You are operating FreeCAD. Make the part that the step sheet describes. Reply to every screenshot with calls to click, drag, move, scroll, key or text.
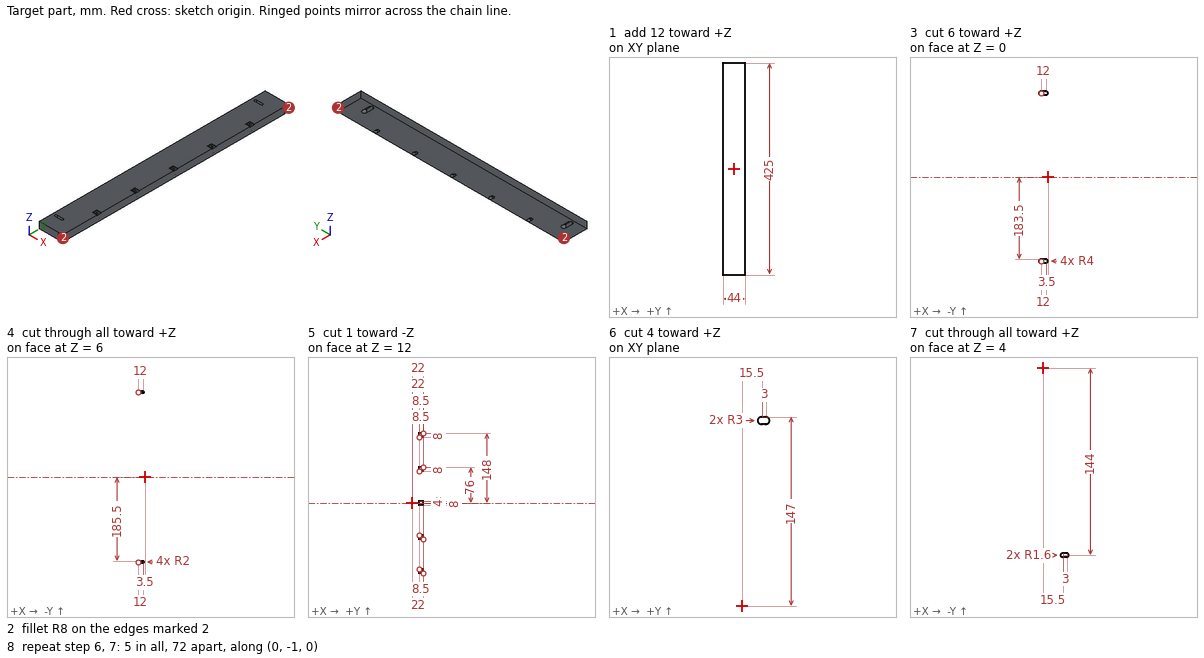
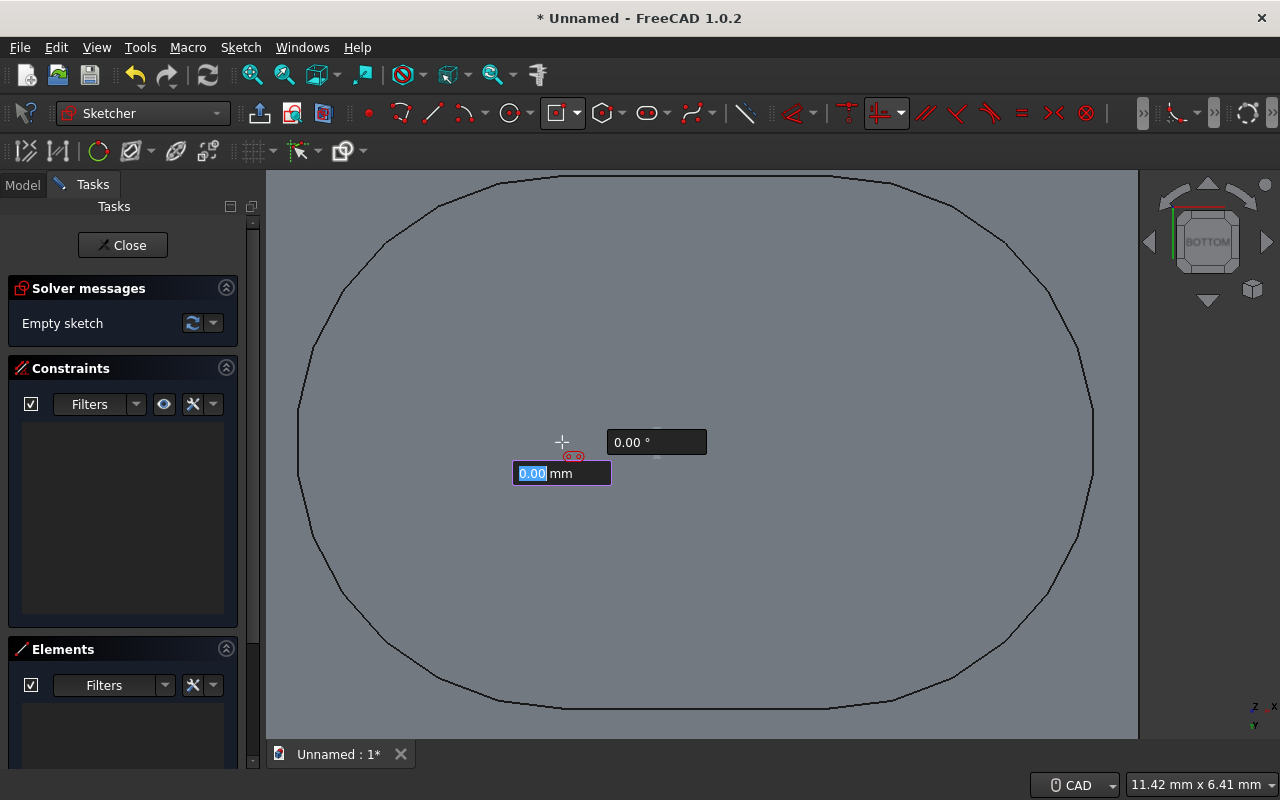
click(829, 442)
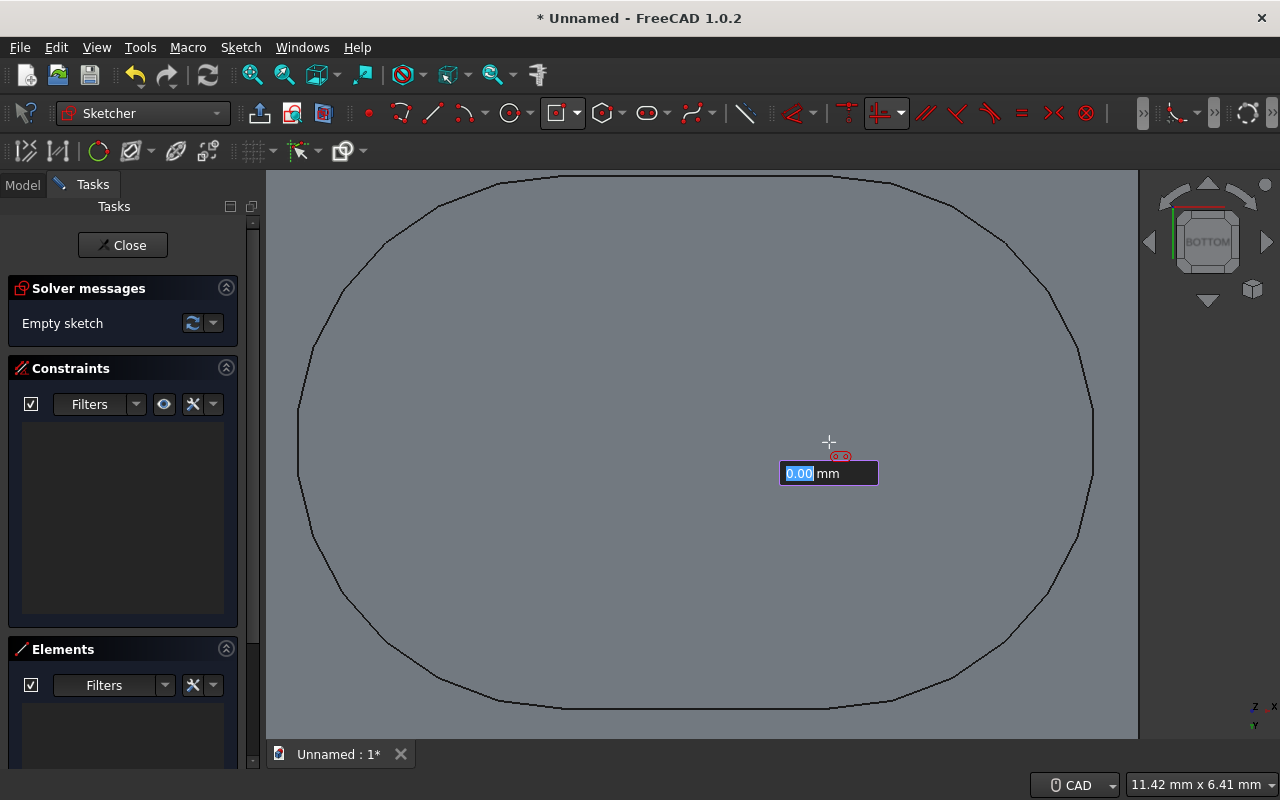
click(695, 584)
key(Escape)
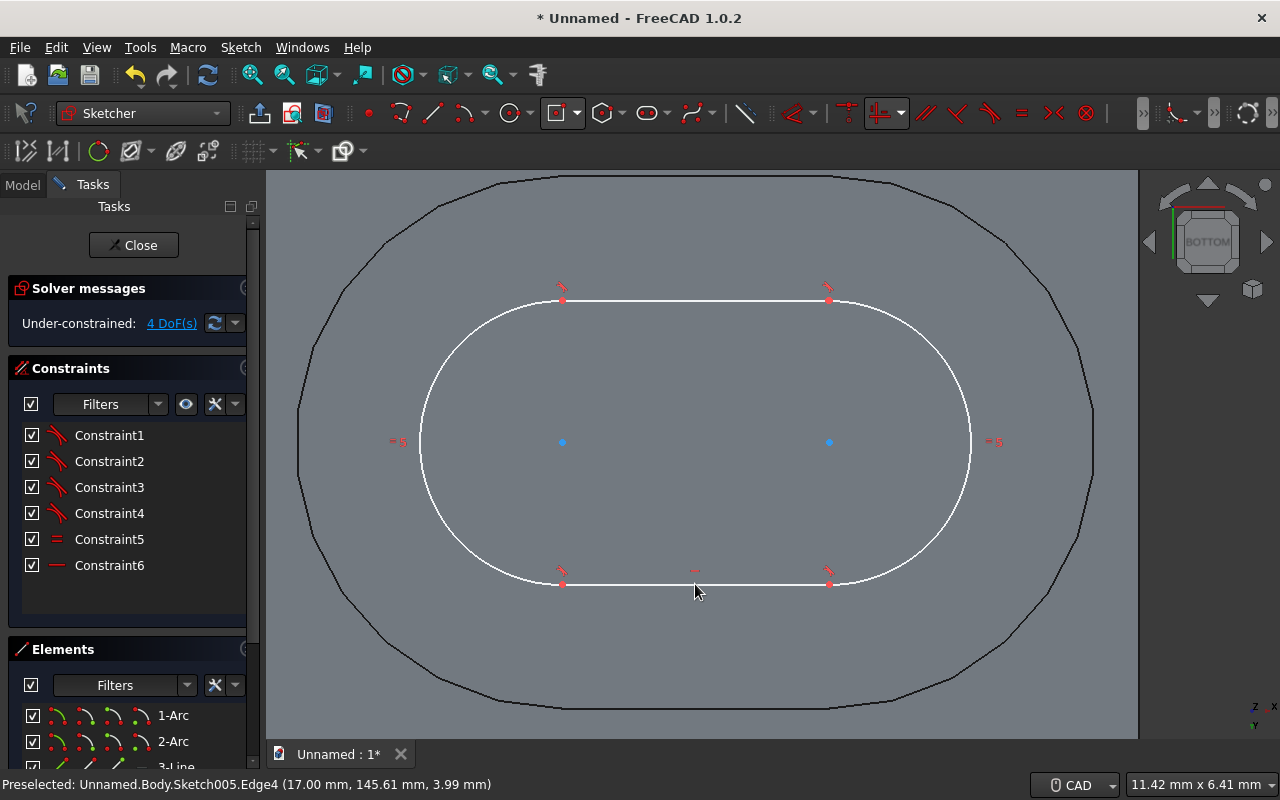
click(792, 114)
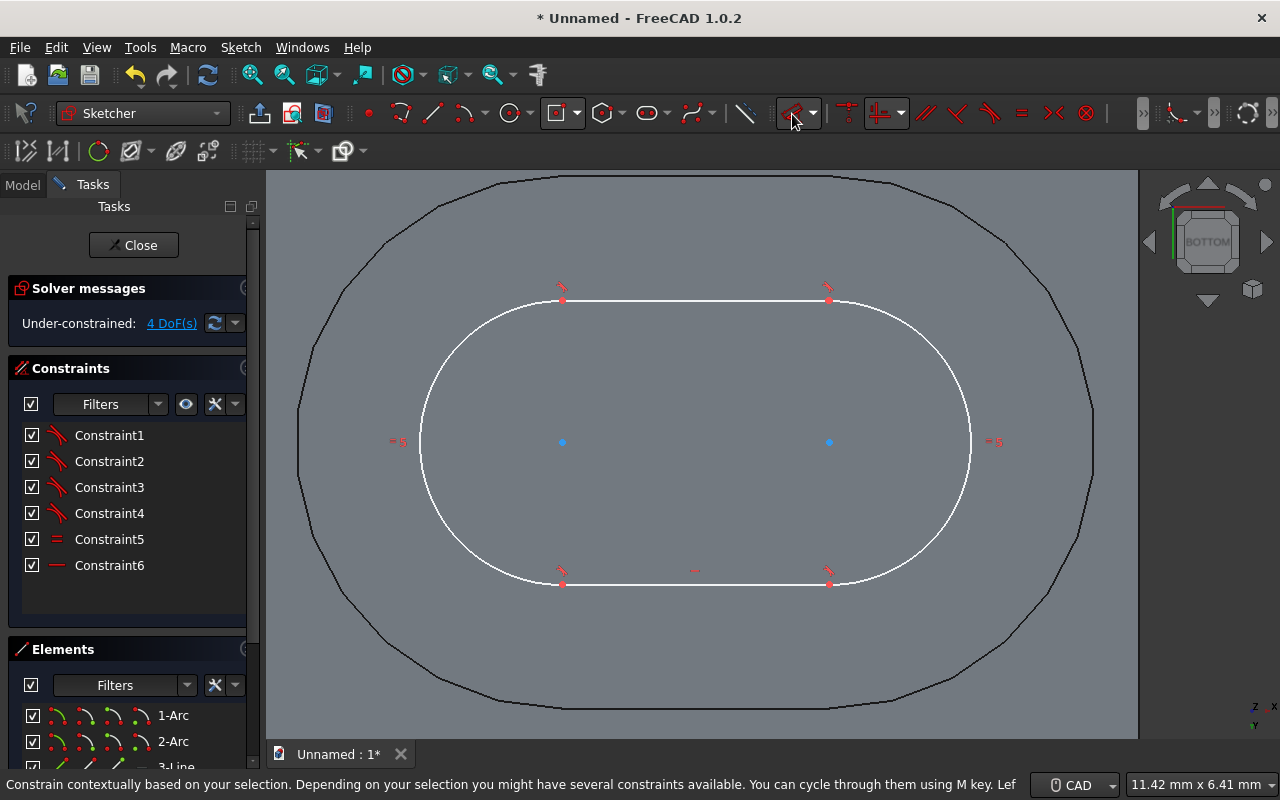
click(447, 360)
click(421, 341)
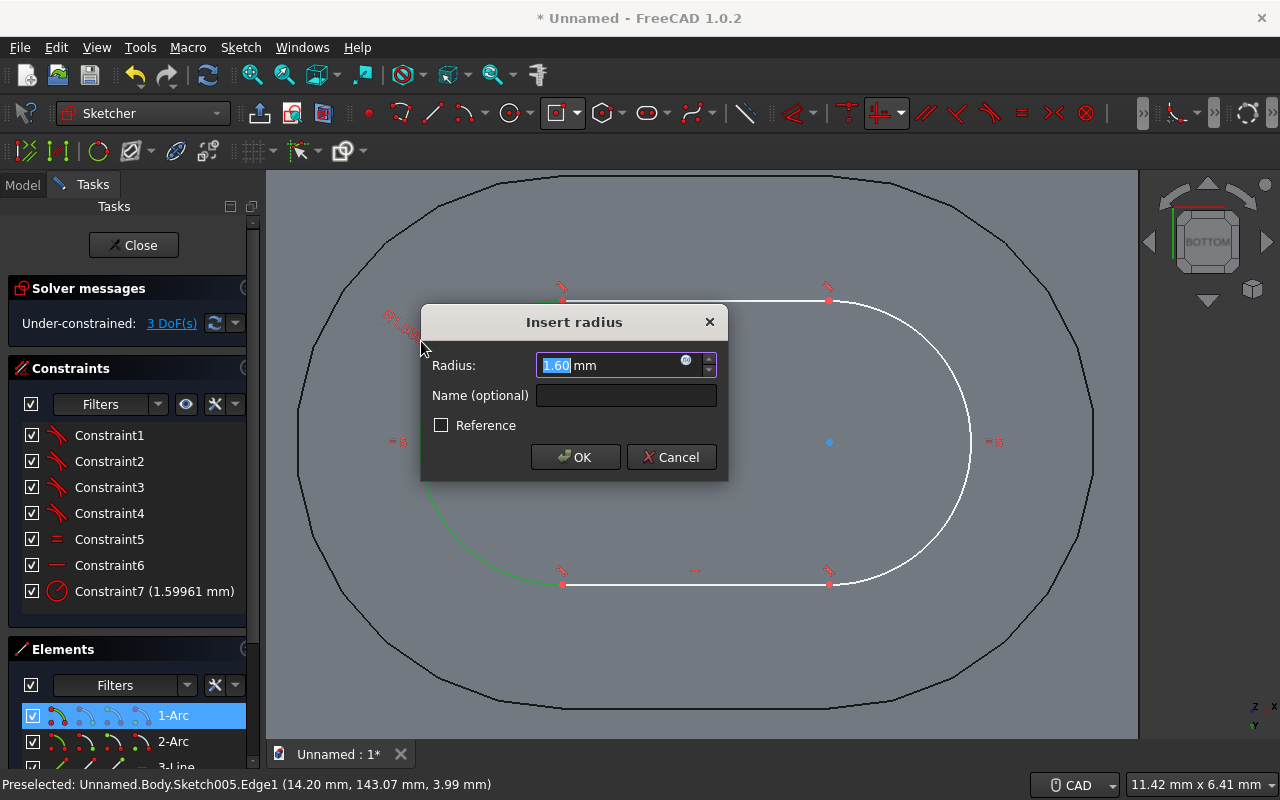
text(1.6)
key(Return)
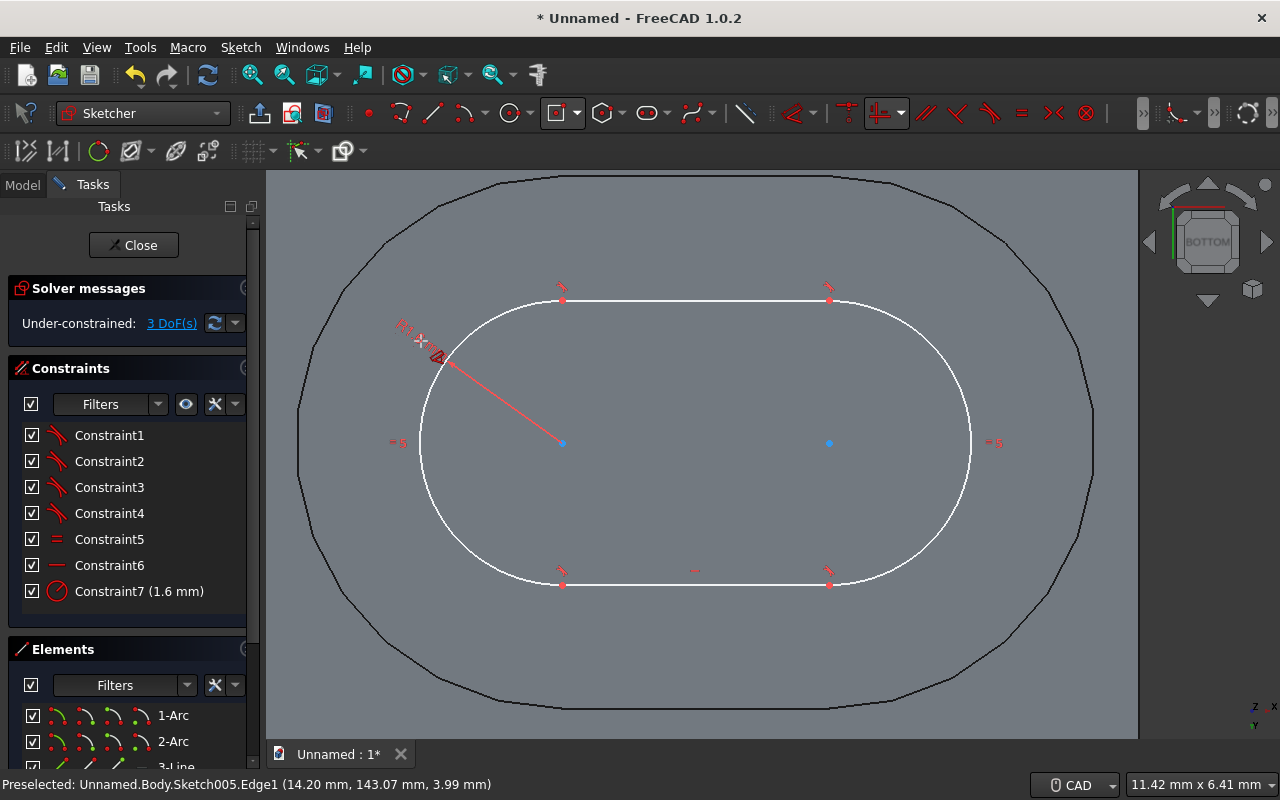
click(642, 301)
click(695, 267)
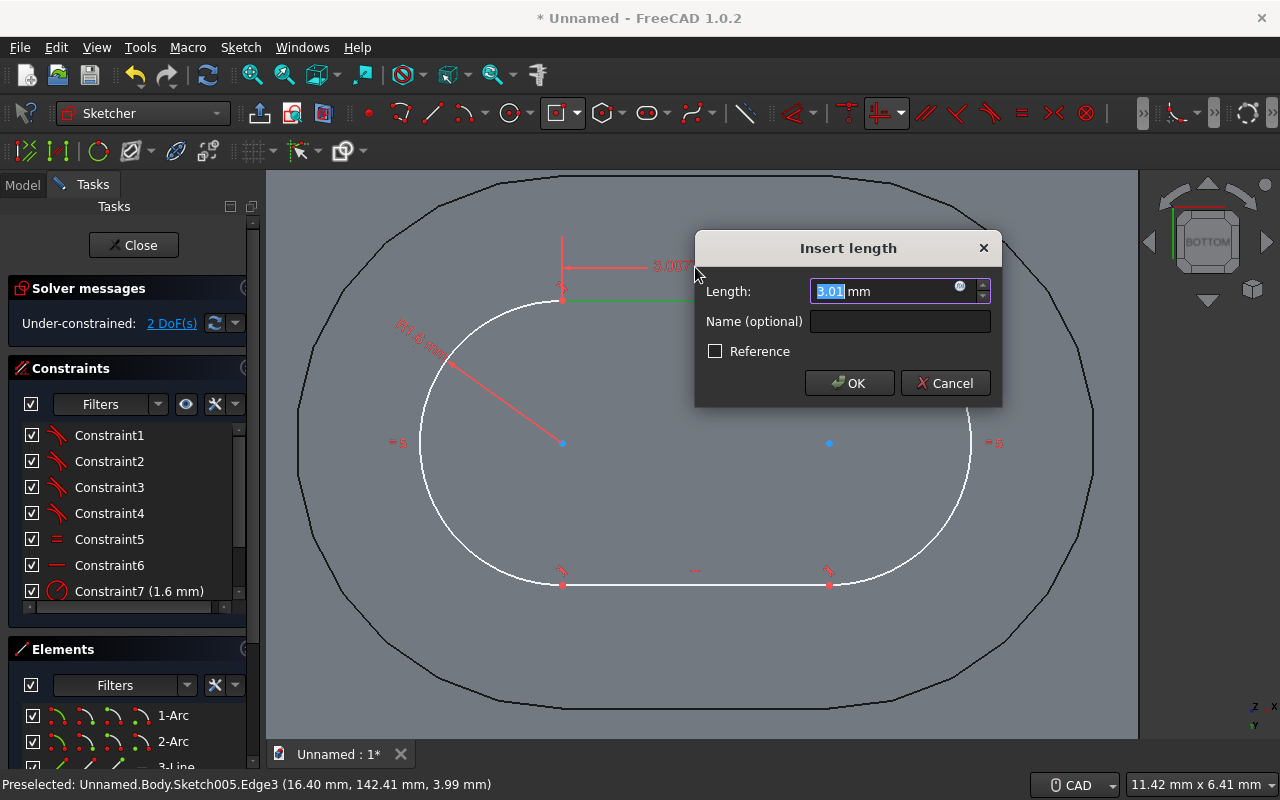
text(3)
key(Return)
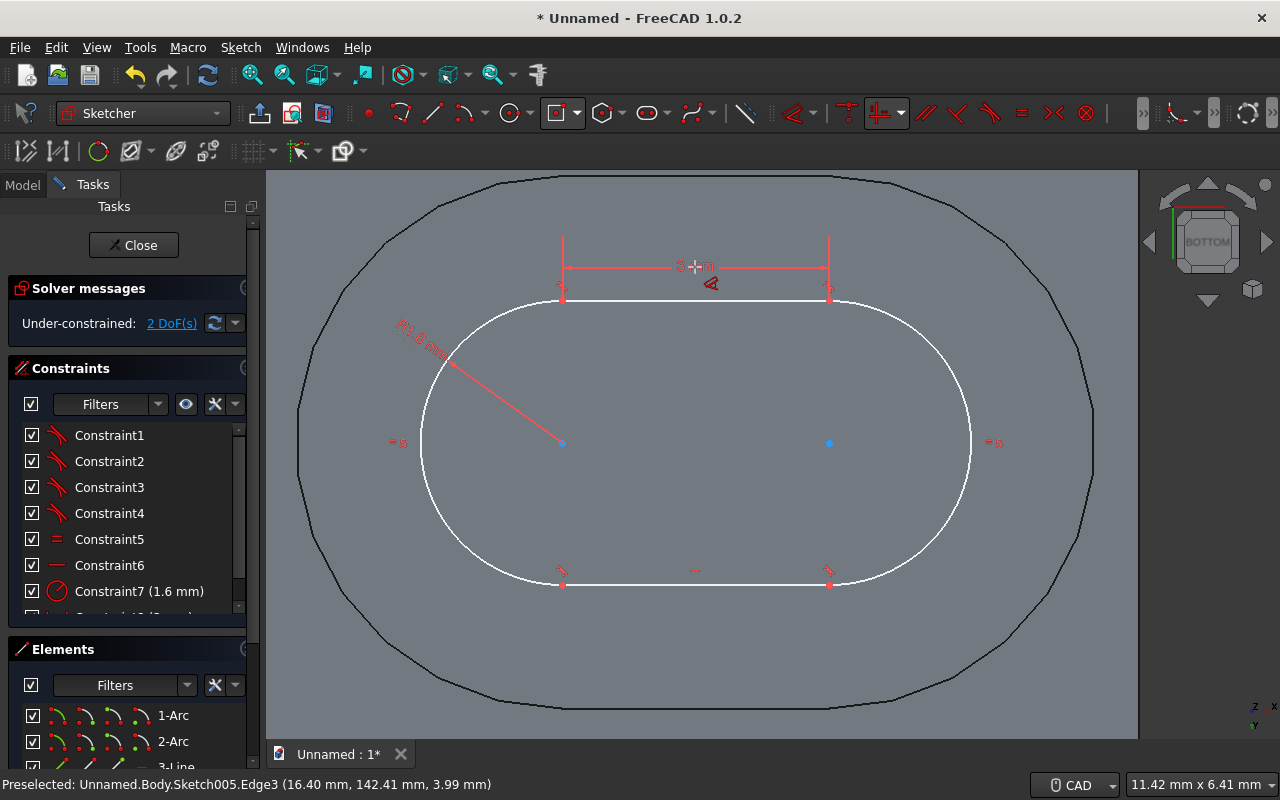
click(563, 443)
click(597, 321)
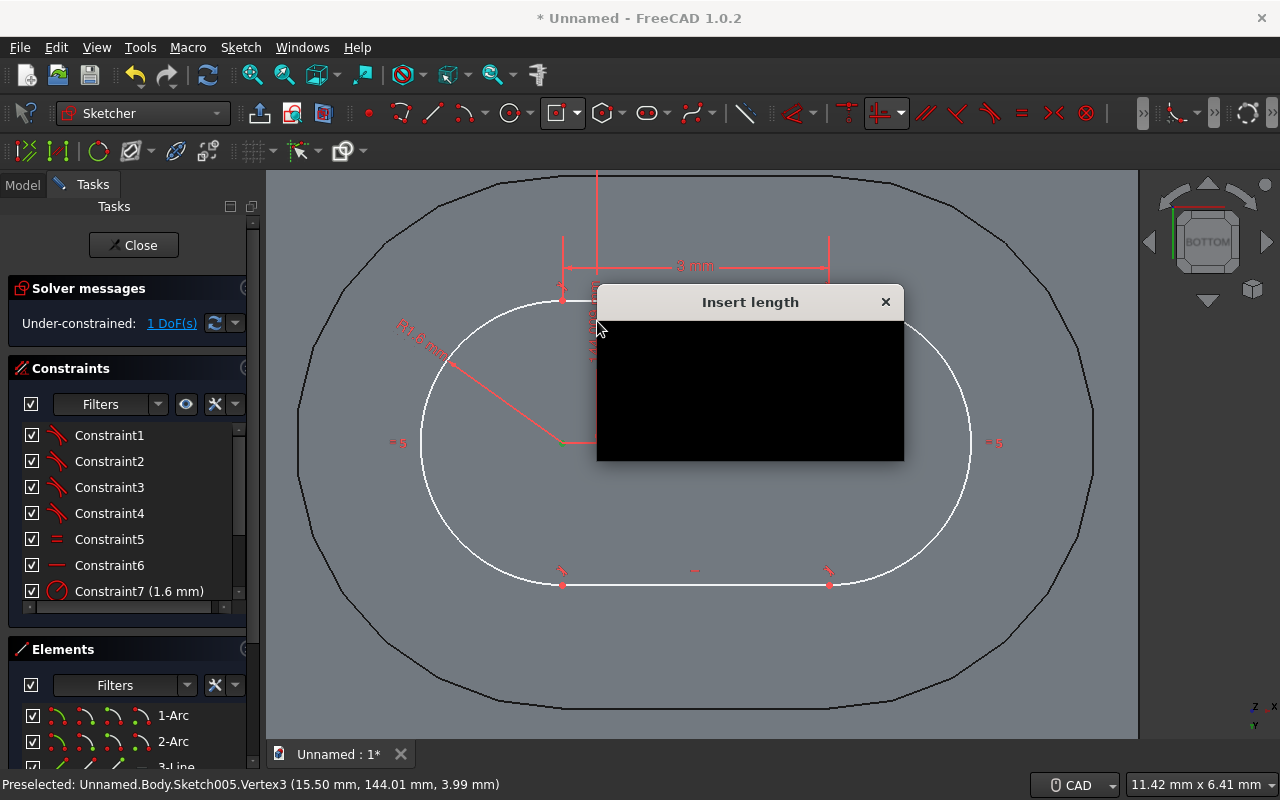
text(144)
key(Return)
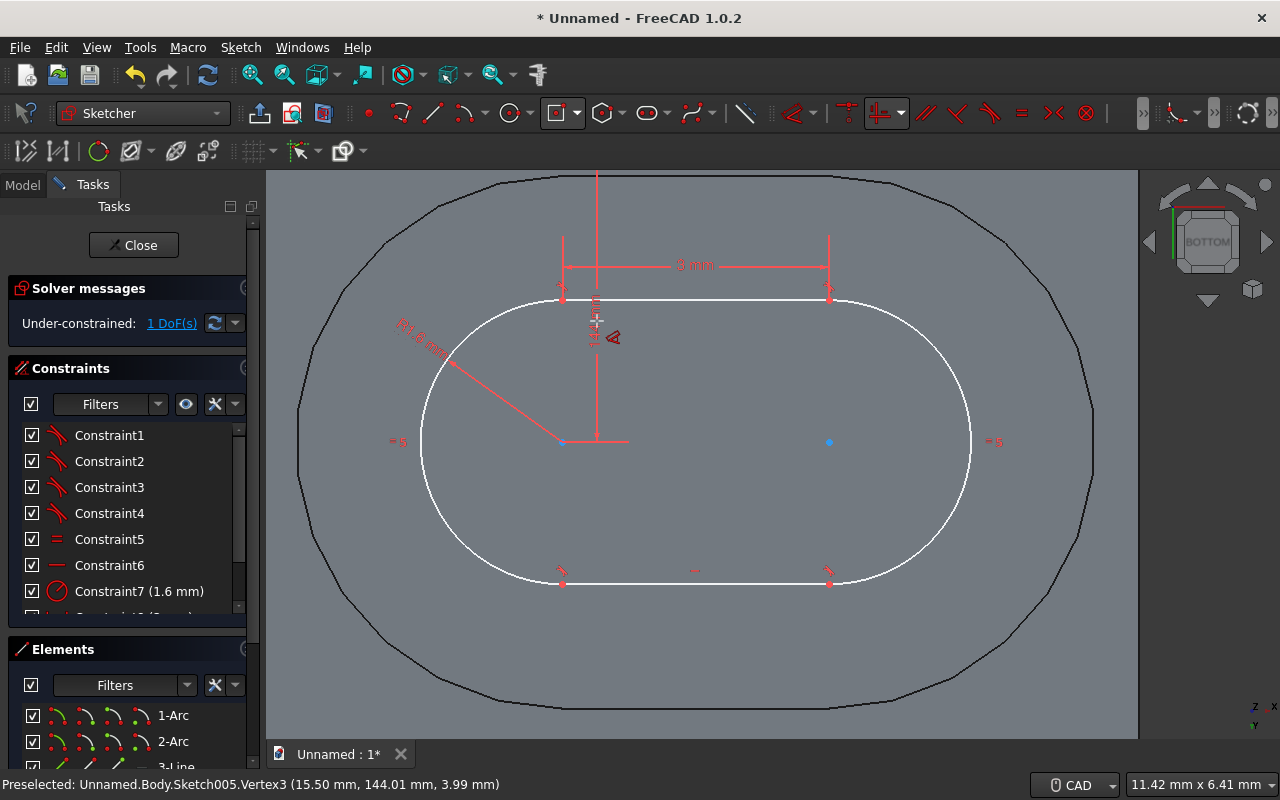
click(563, 300)
click(334, 334)